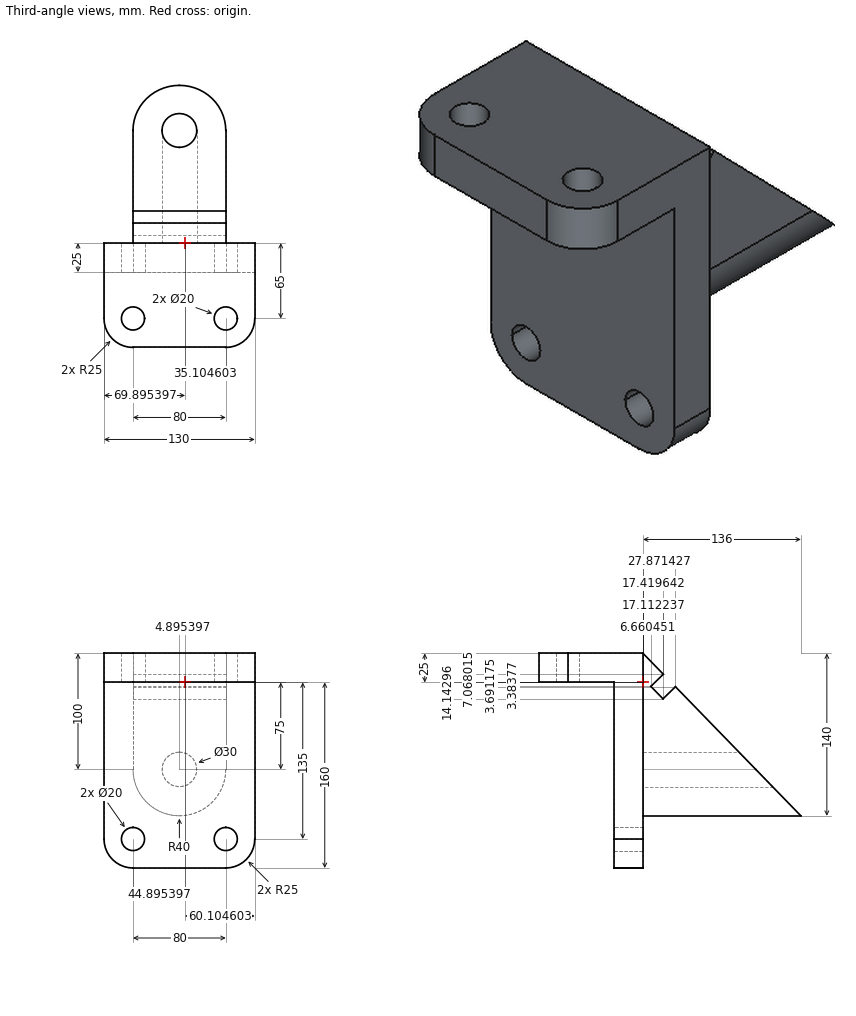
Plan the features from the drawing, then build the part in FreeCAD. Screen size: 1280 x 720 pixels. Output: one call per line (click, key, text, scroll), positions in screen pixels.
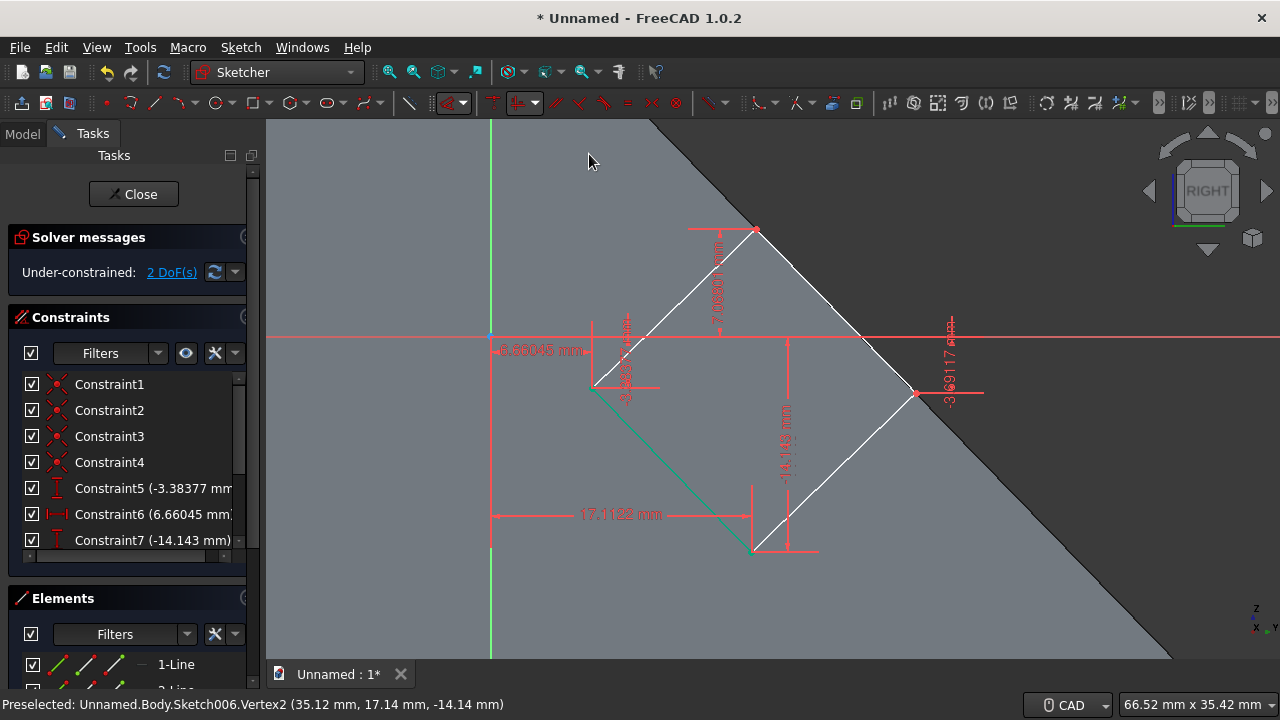
click(916, 393)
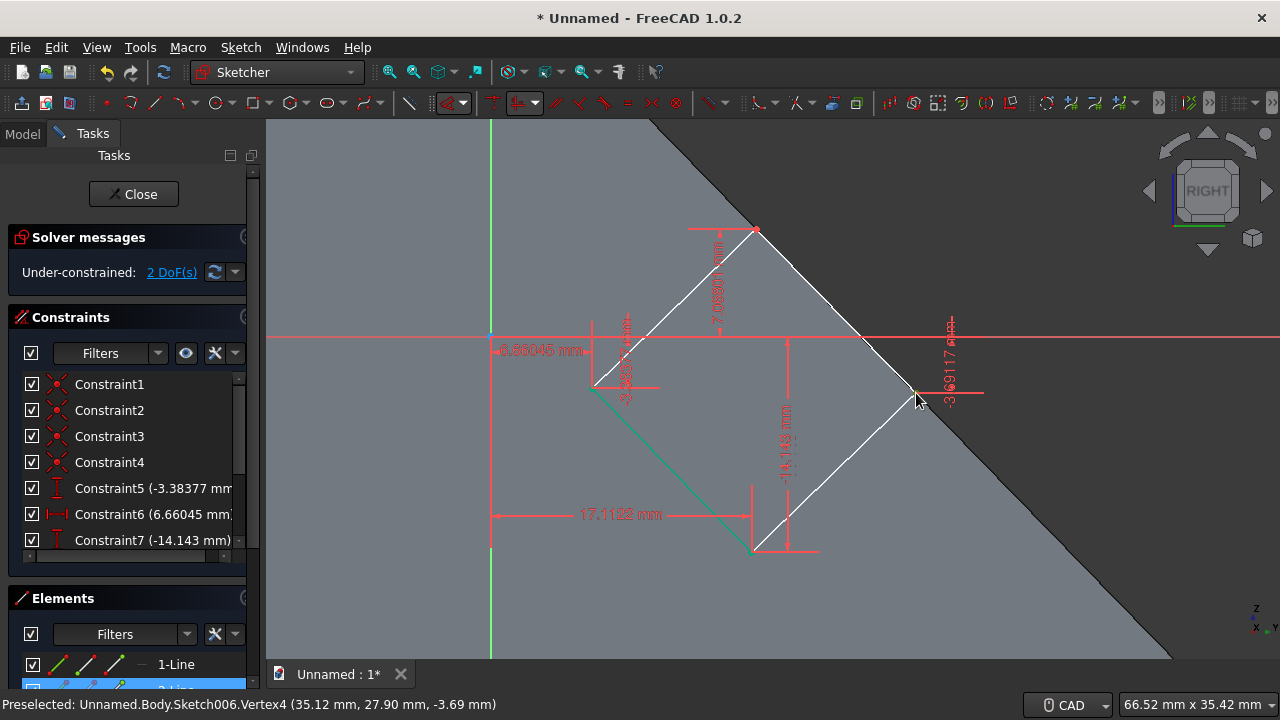
click(466, 104)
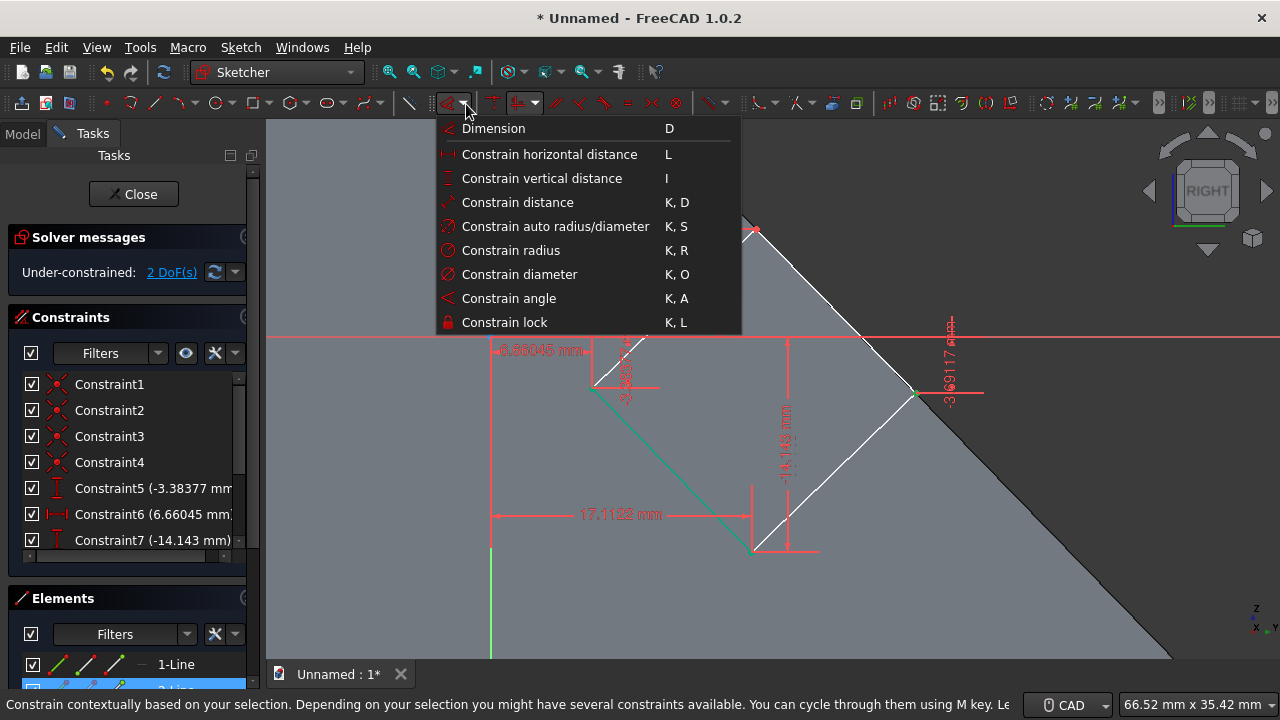
click(589, 154)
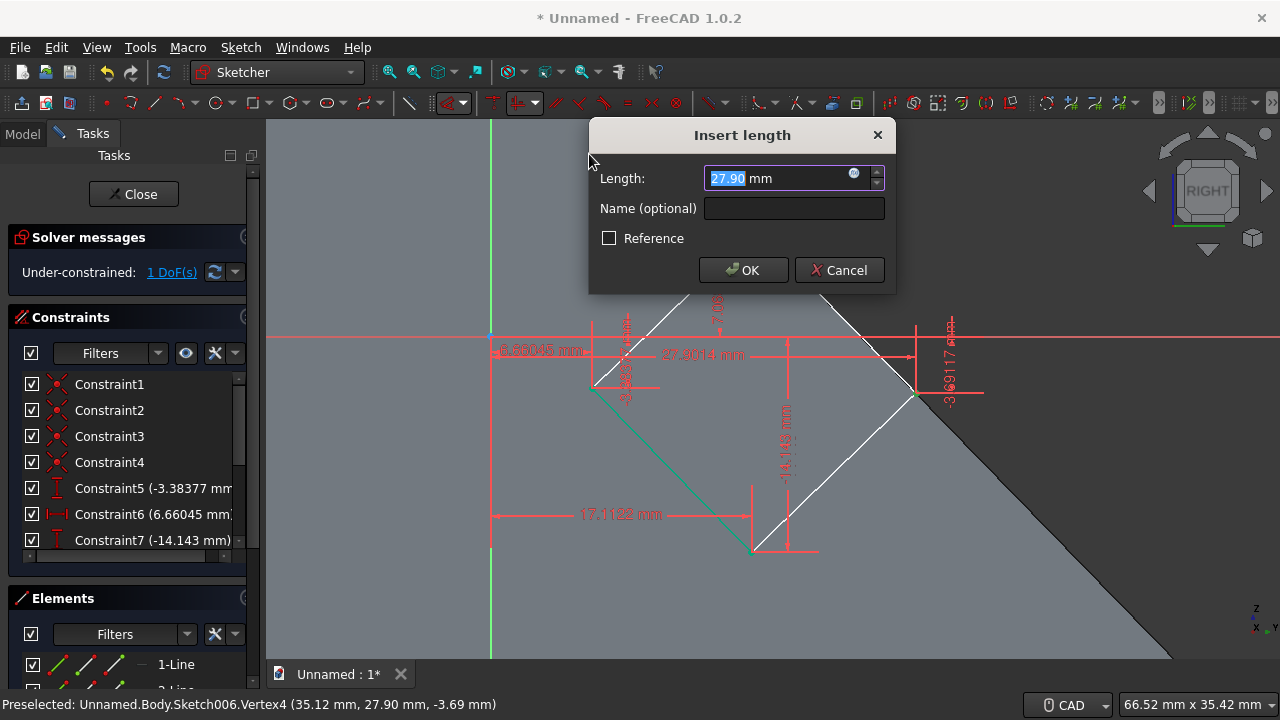
text(27.871427)
key(Return)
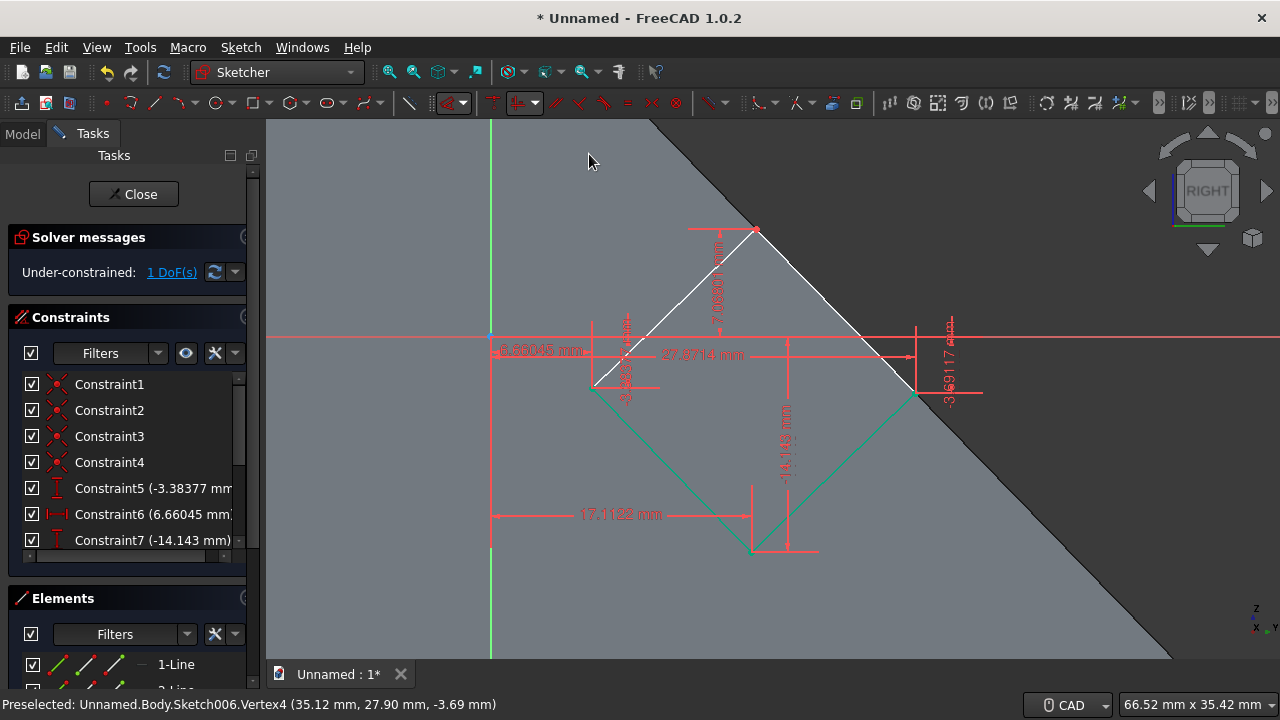
click(756, 229)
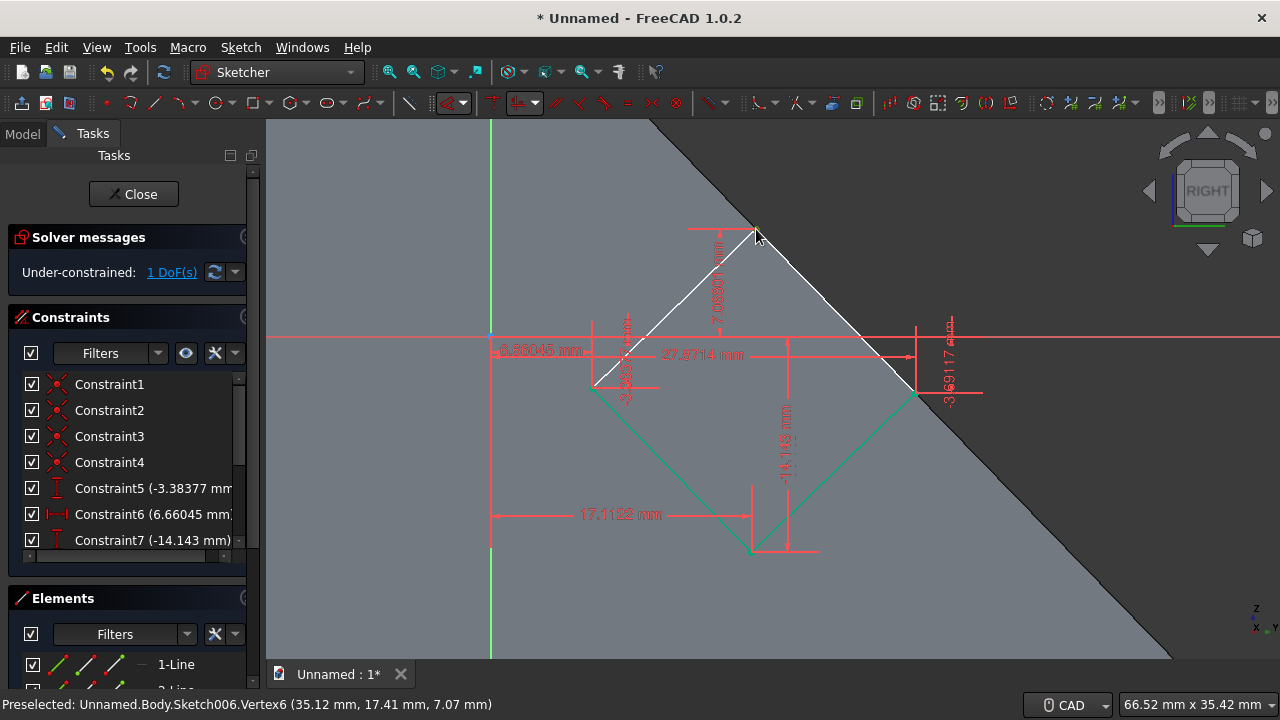
key(l)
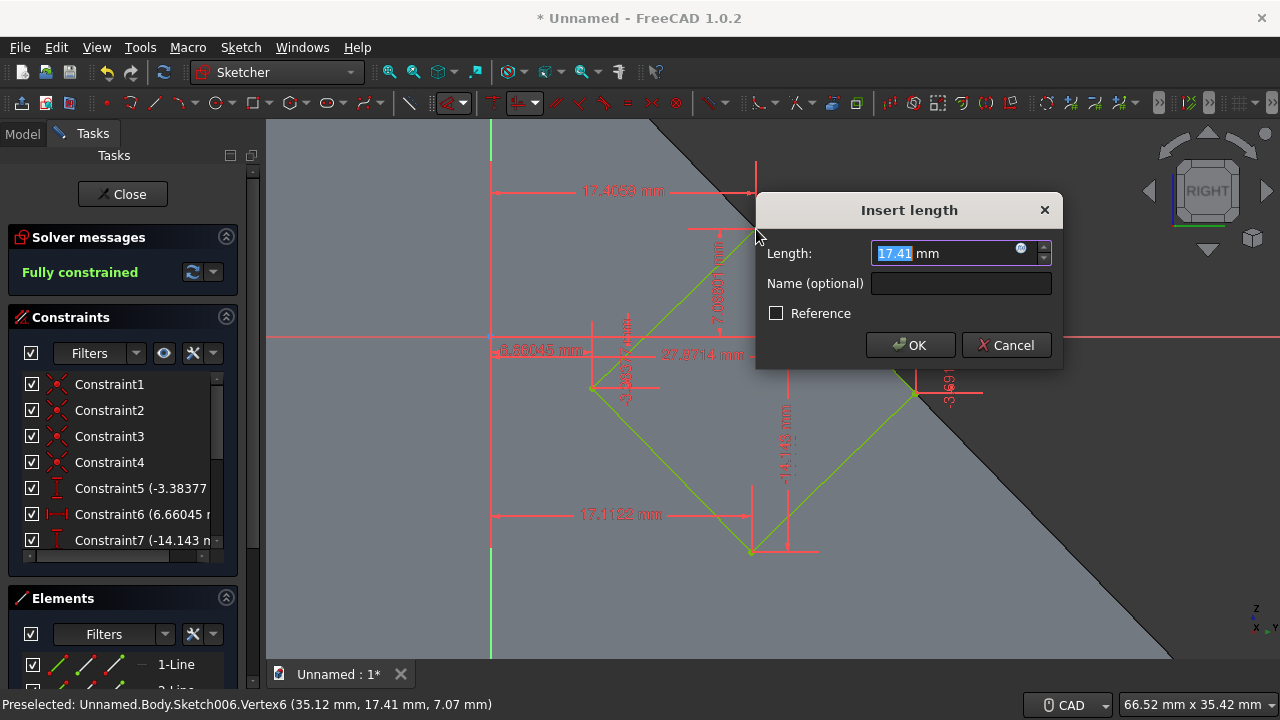
text(17.419642)
key(Return)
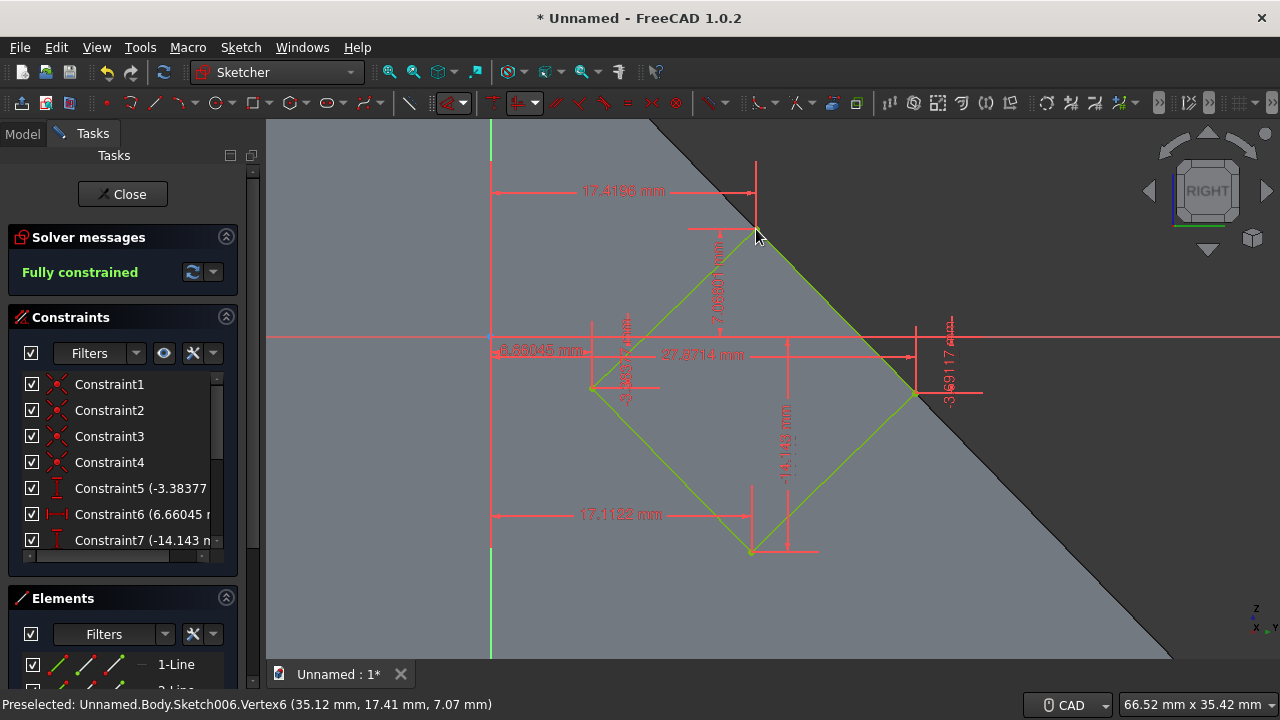
click(123, 194)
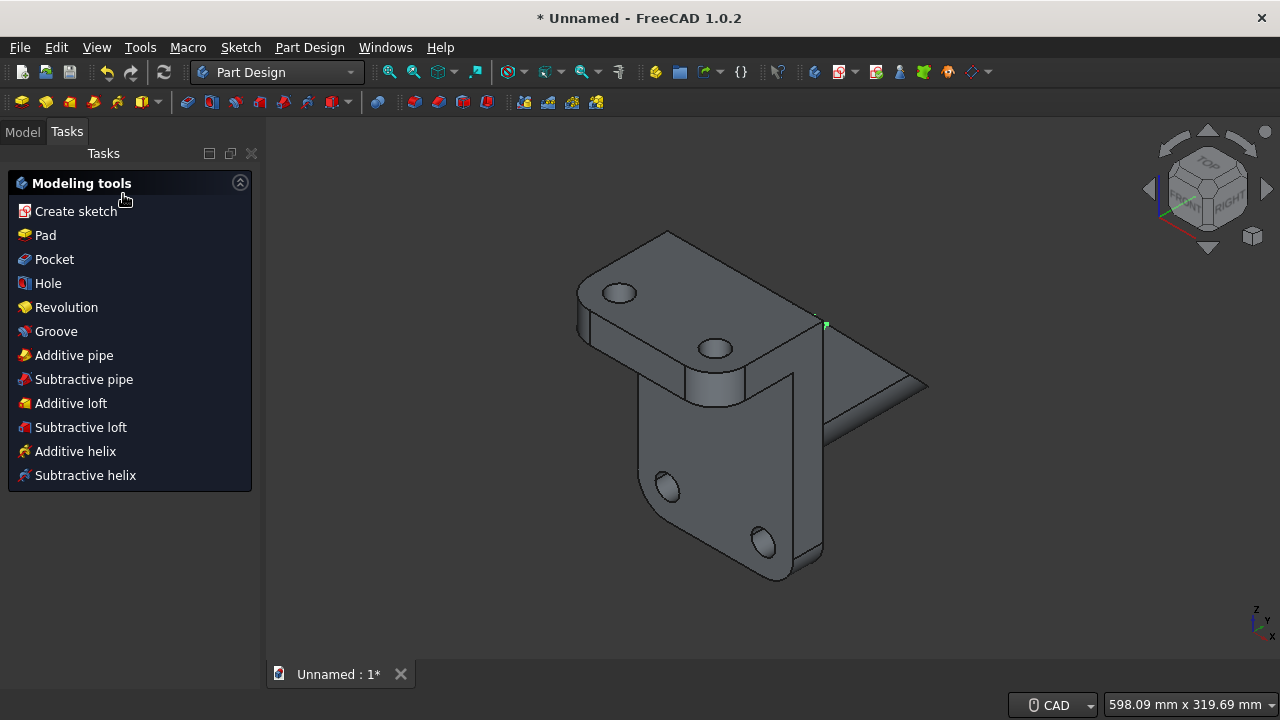
click(188, 102)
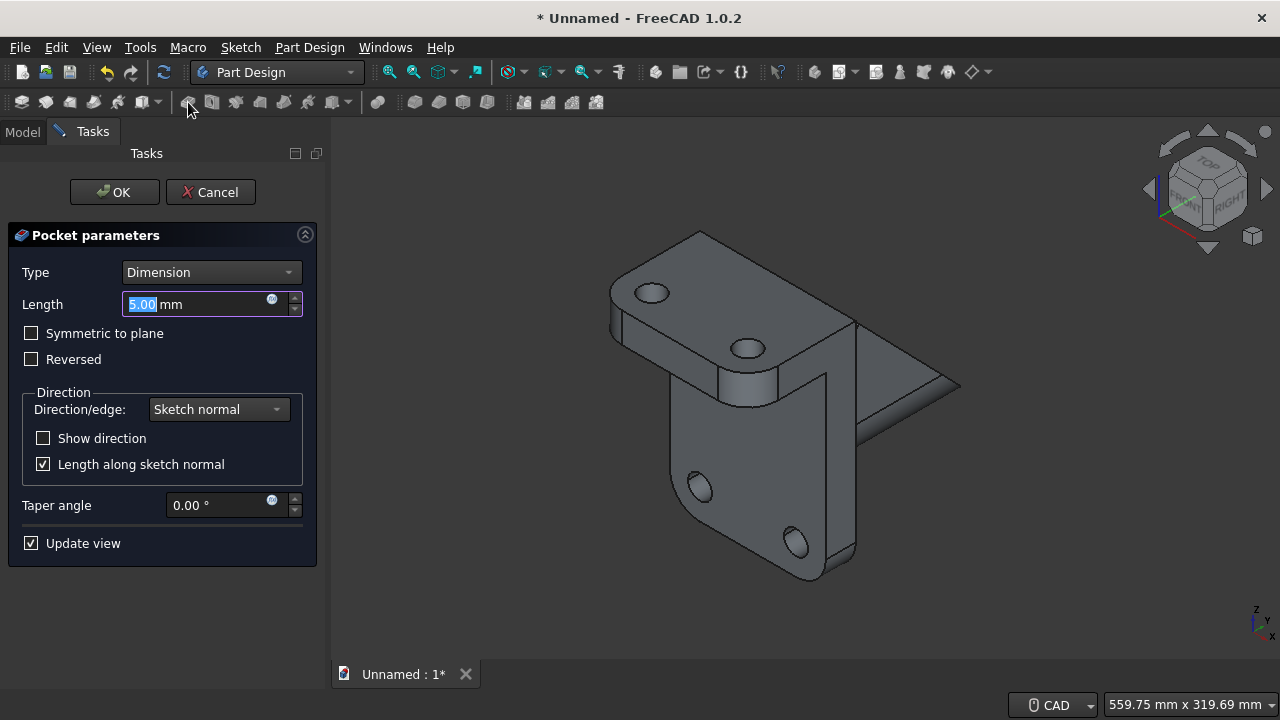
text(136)
key(Tab)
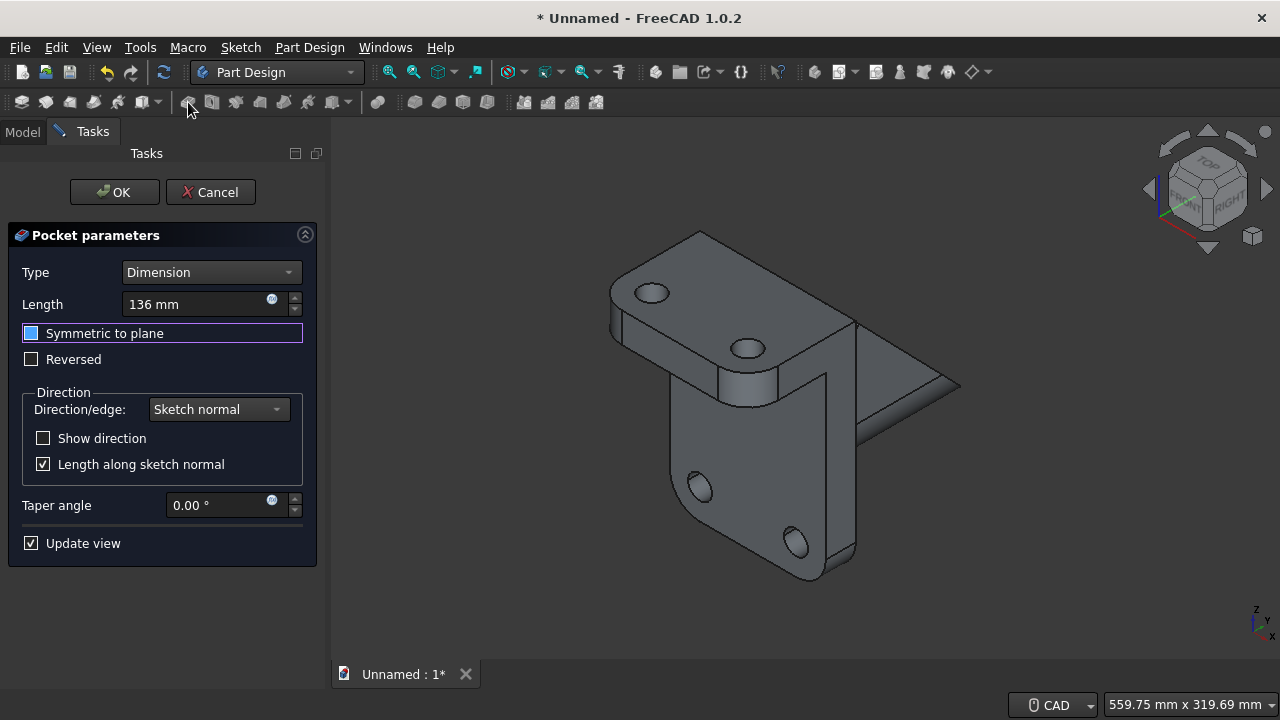
click(115, 192)